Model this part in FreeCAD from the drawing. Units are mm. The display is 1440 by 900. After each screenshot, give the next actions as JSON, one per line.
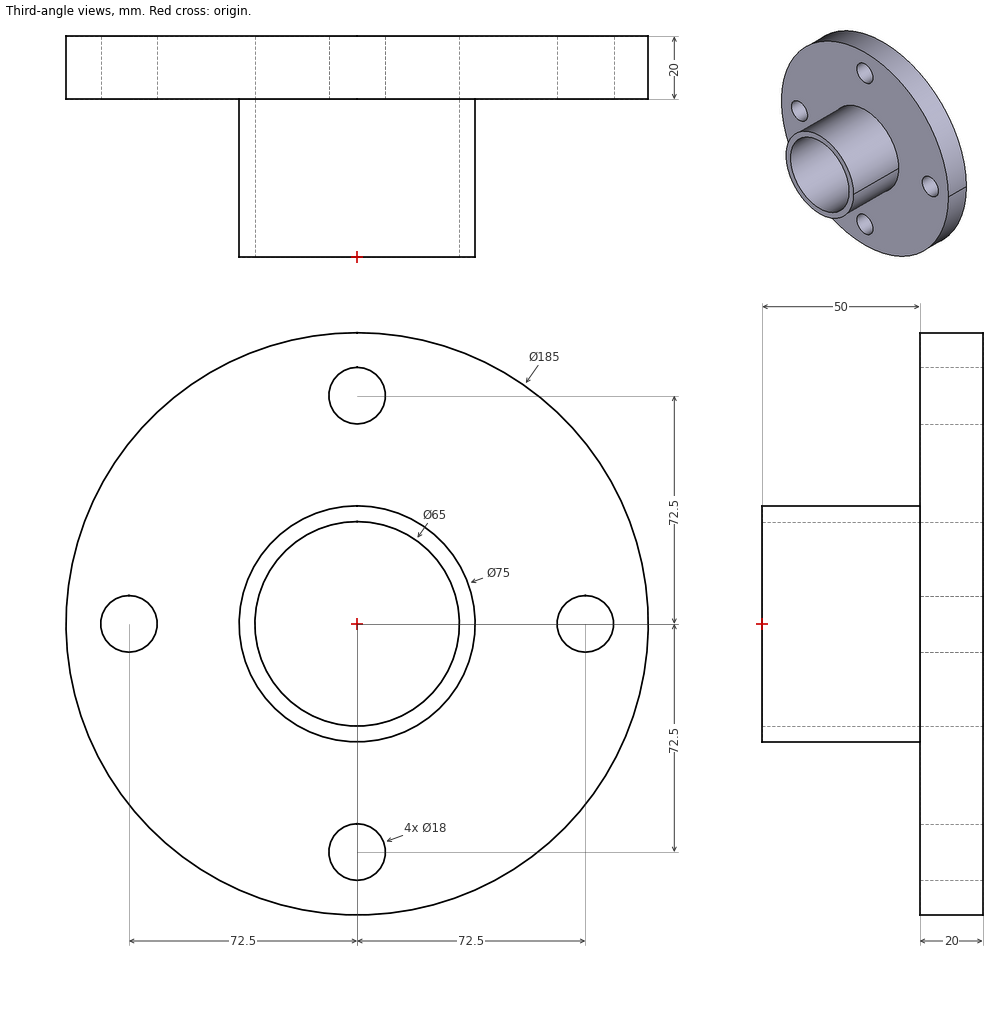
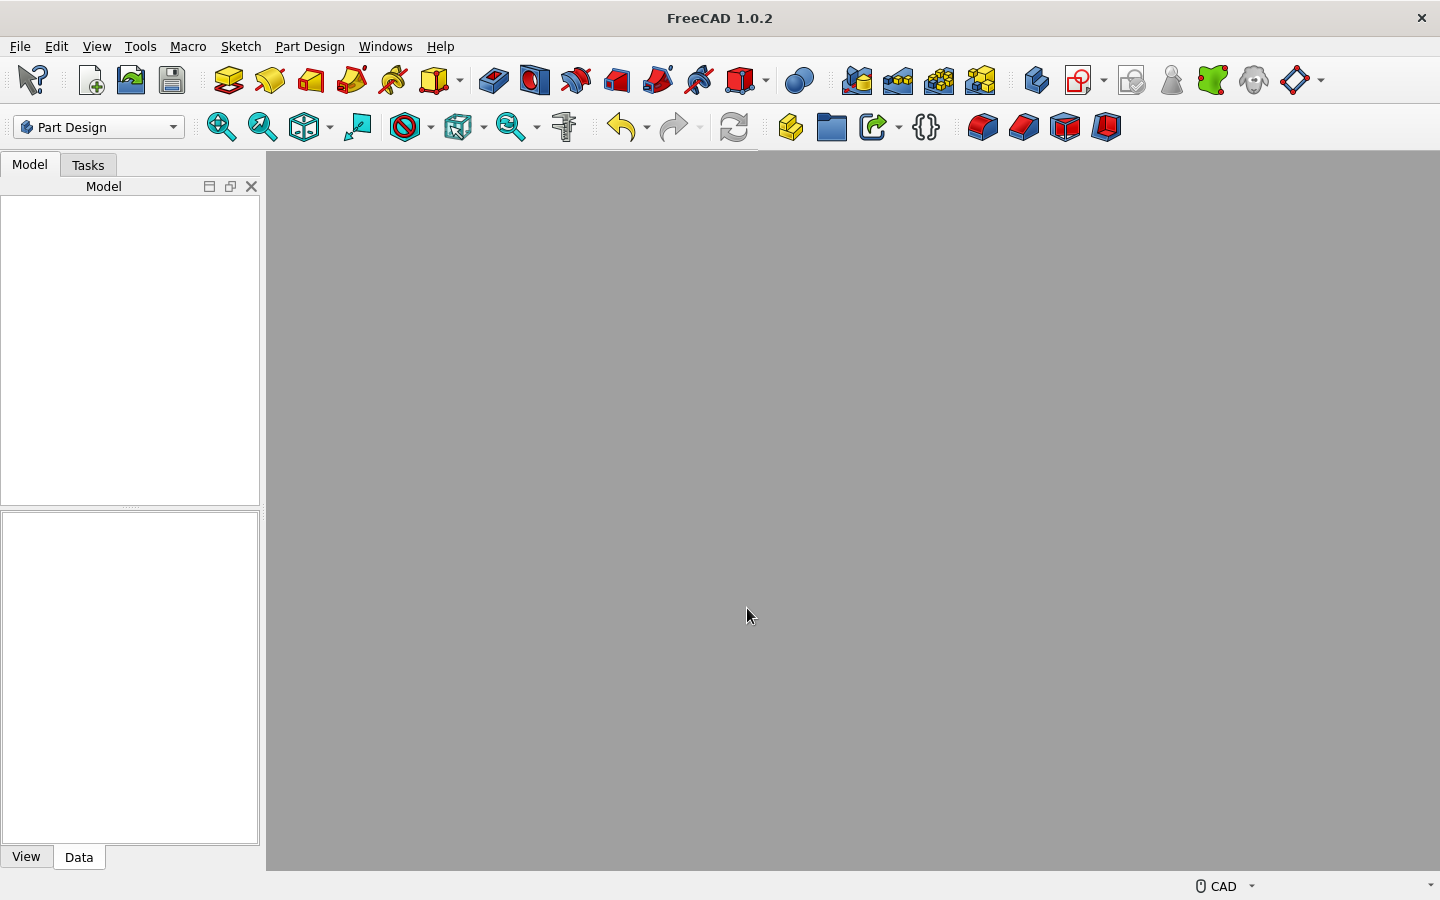
{"action": "key", "text": "ctrl+n"}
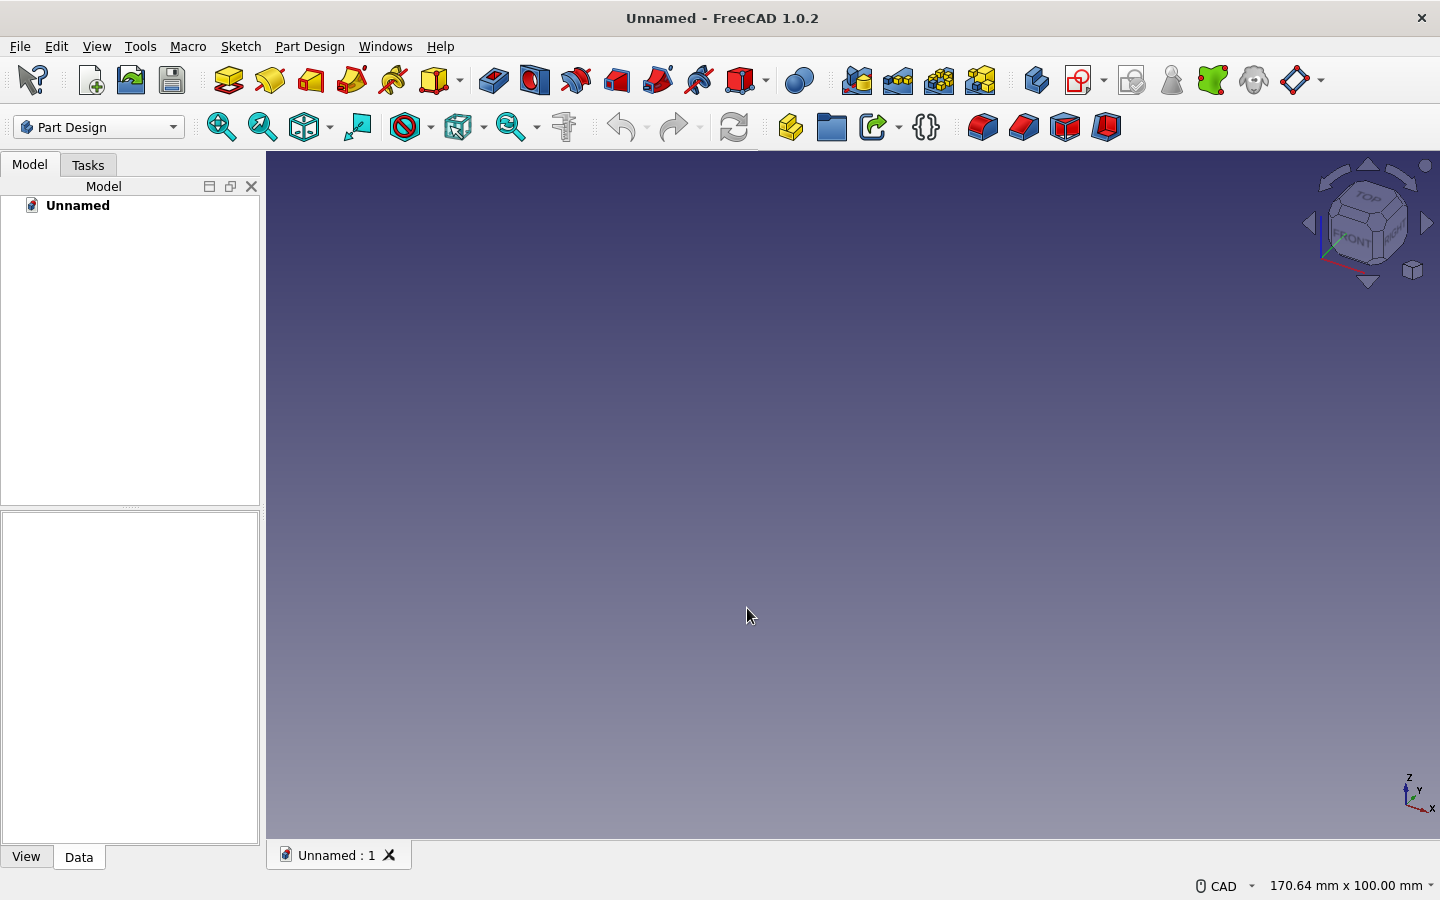
{"action": "left_click", "coordinate": [1078, 80]}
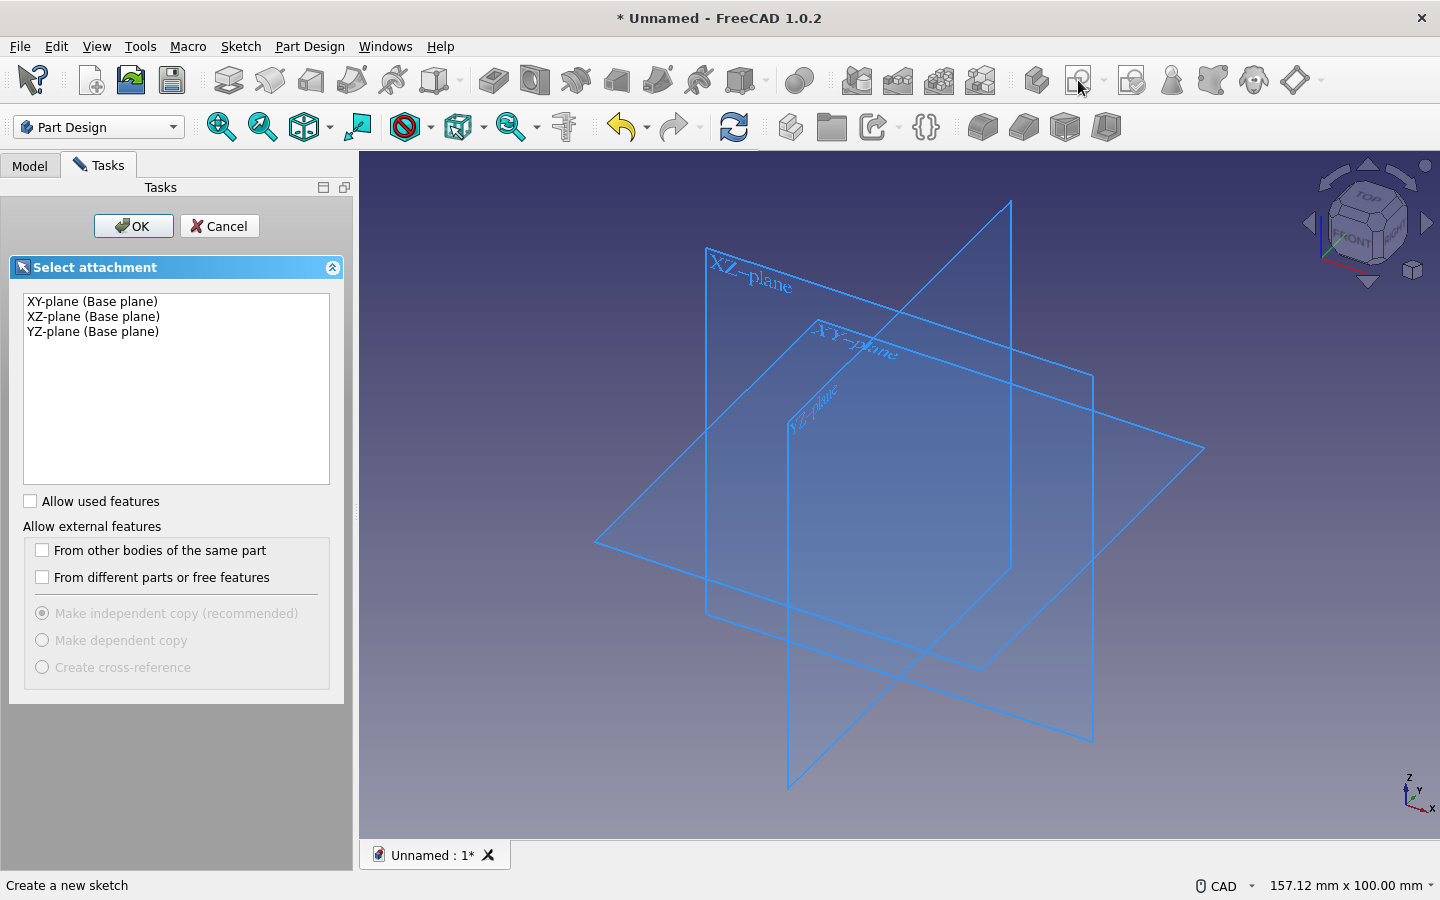
{"action": "left_click", "coordinate": [84, 316]}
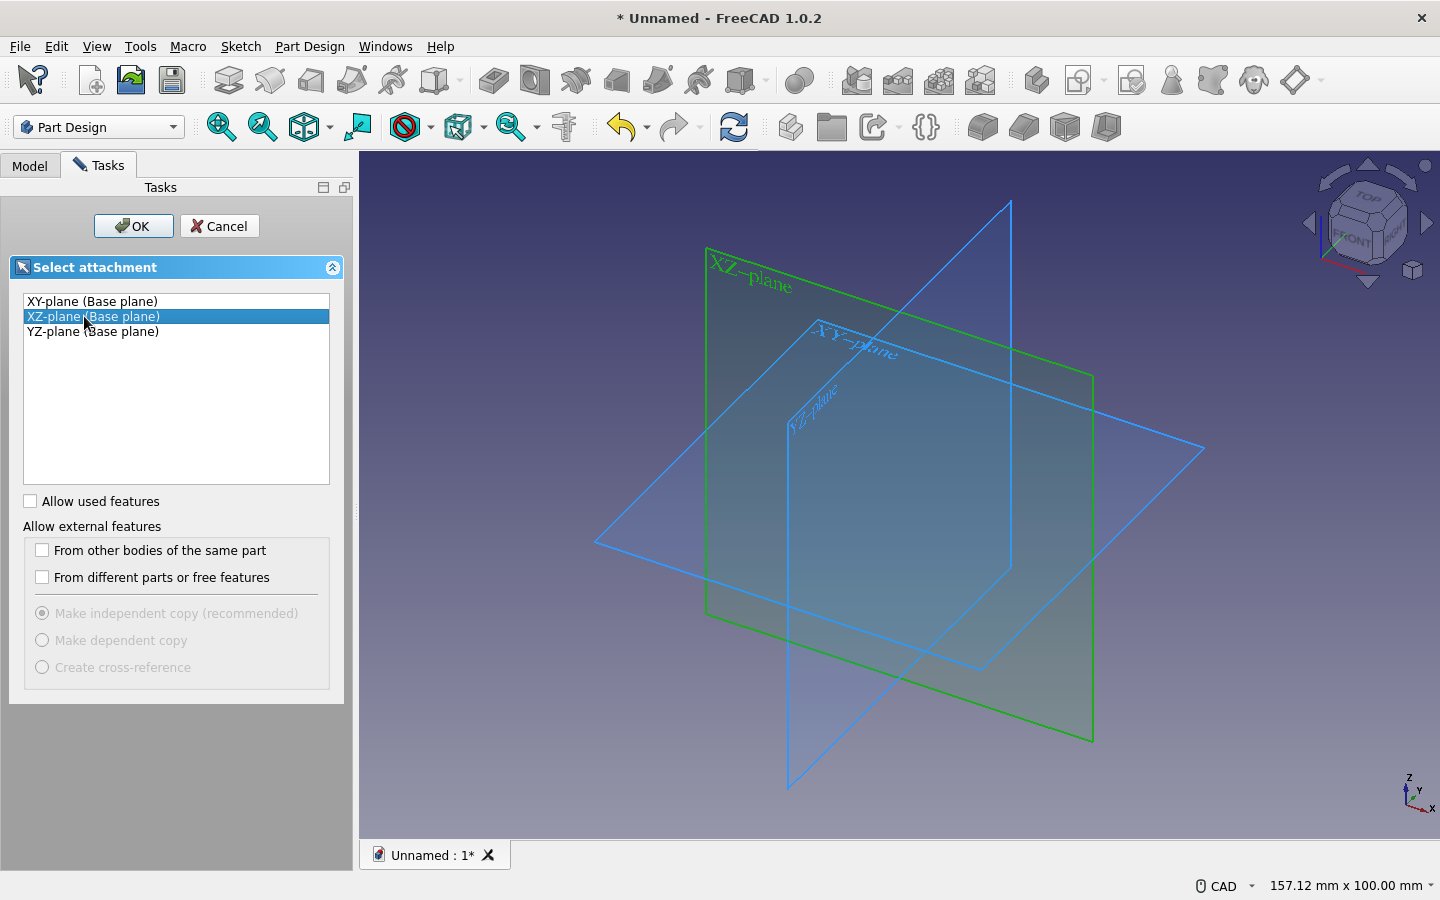
{"action": "left_click", "coordinate": [134, 226]}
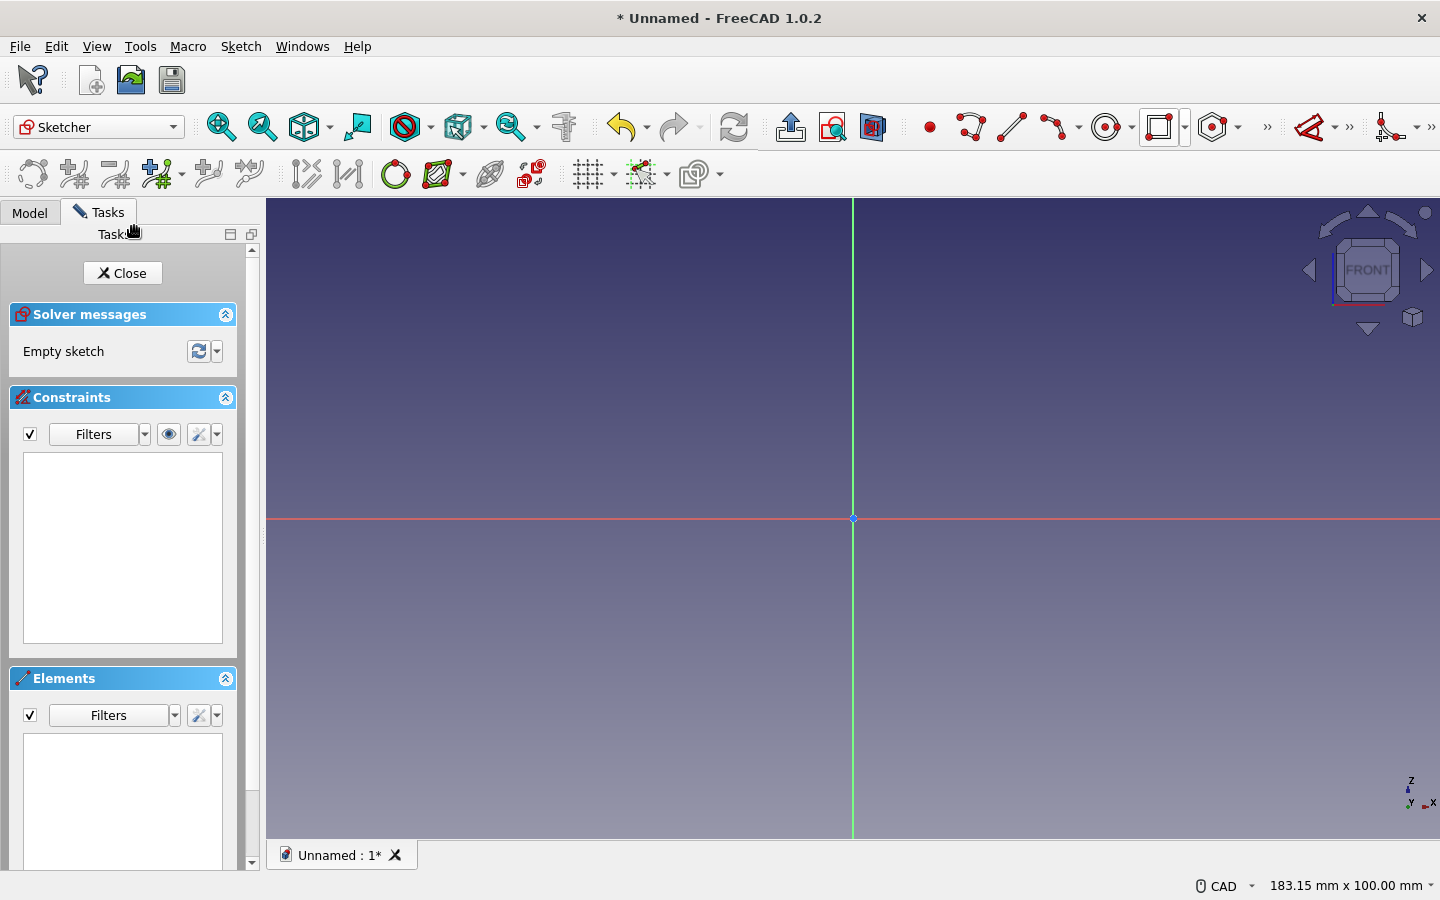
{"action": "key", "text": "g c"}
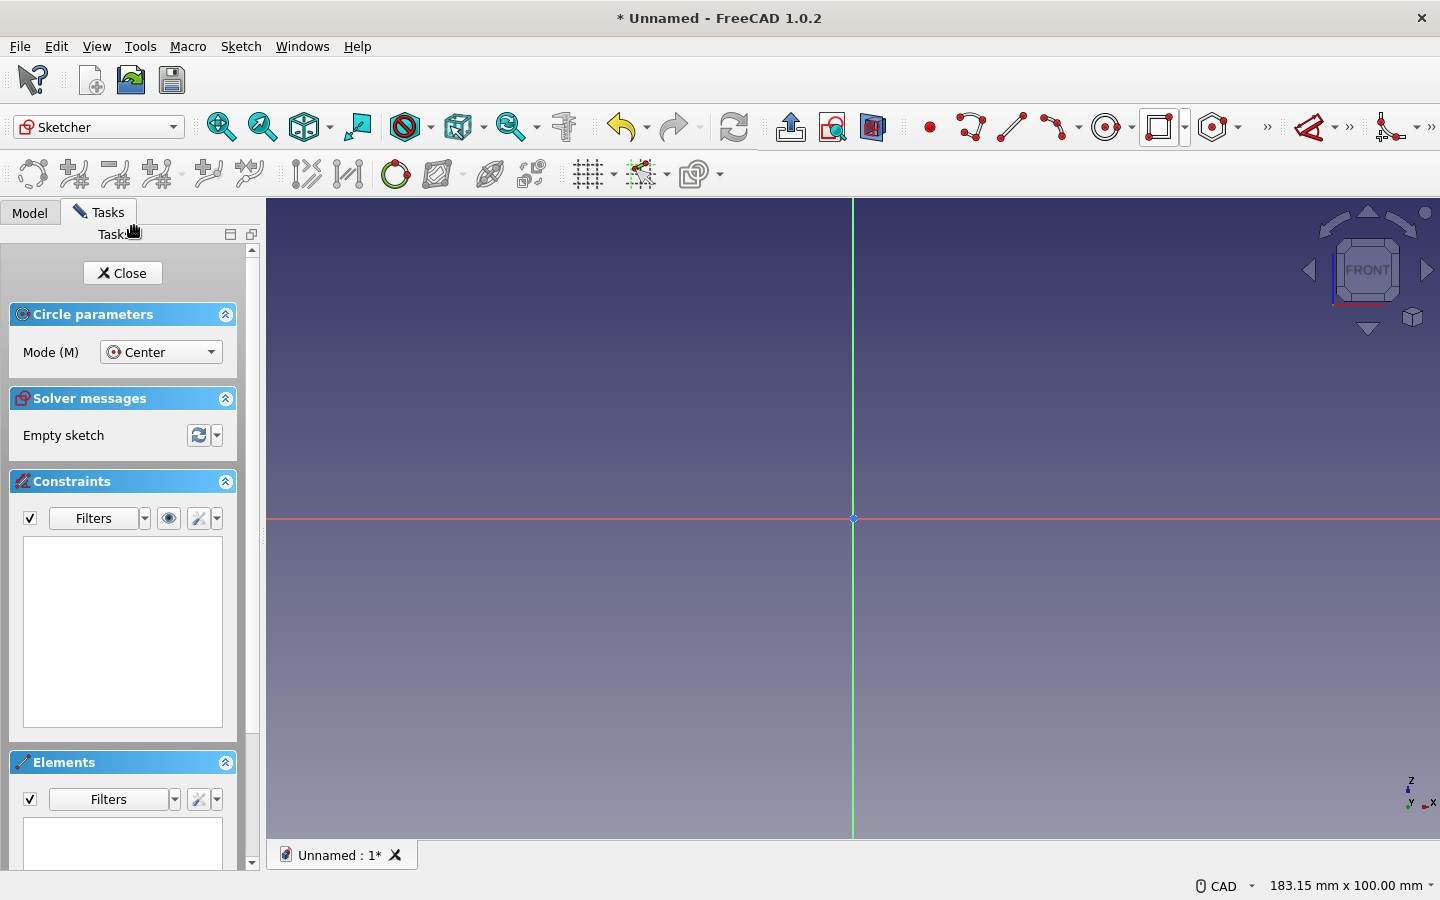
{"action": "left_click", "coordinate": [853, 518]}
{"action": "left_click", "coordinate": [1023, 349]}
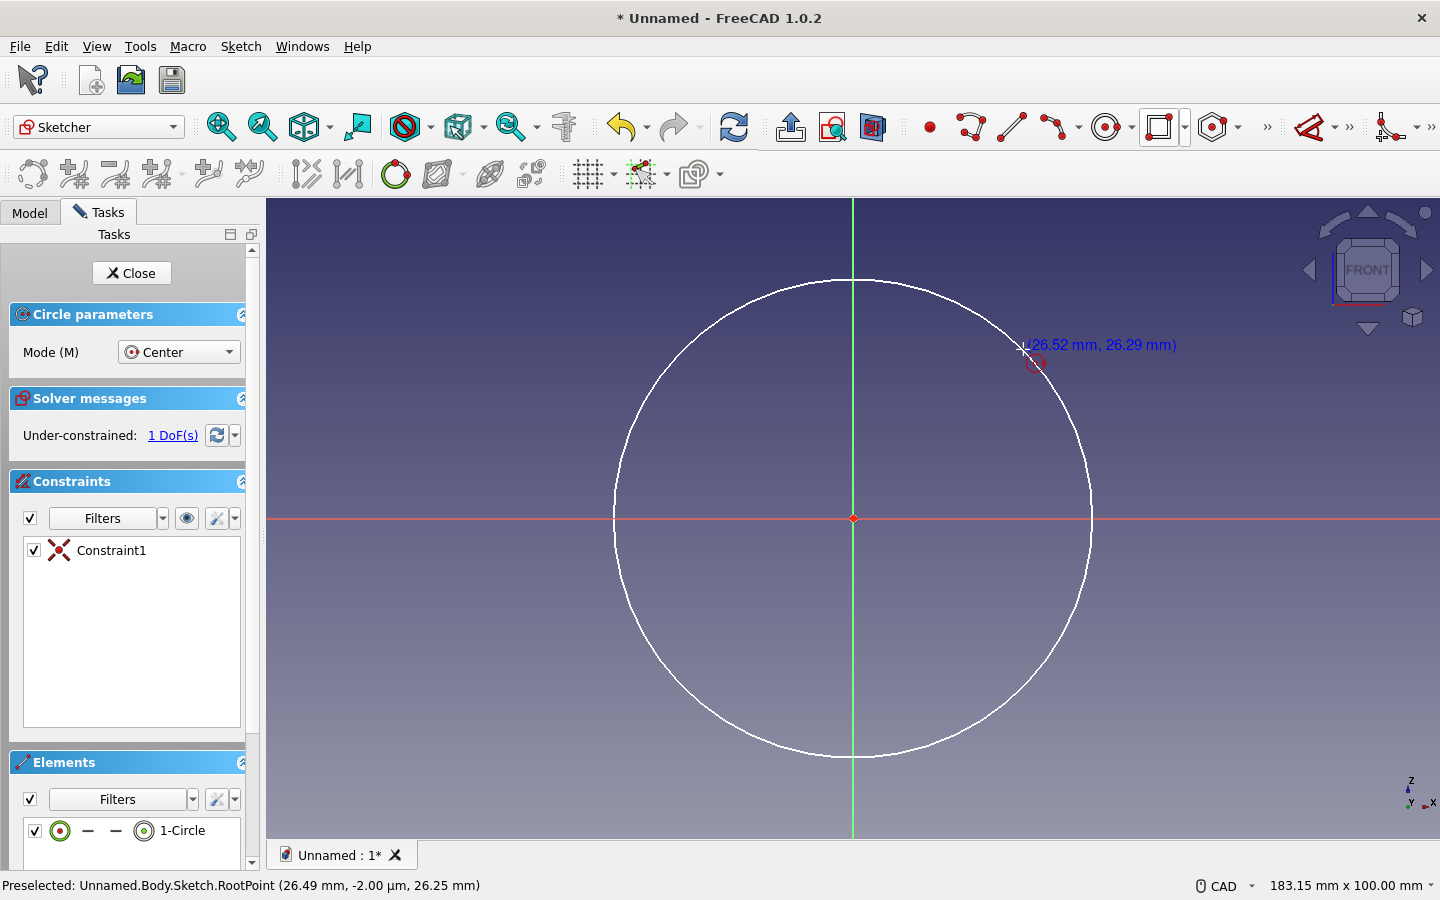
{"action": "left_click", "coordinate": [853, 518]}
{"action": "left_click", "coordinate": [1000, 371]}
{"action": "key", "text": "Escape"}